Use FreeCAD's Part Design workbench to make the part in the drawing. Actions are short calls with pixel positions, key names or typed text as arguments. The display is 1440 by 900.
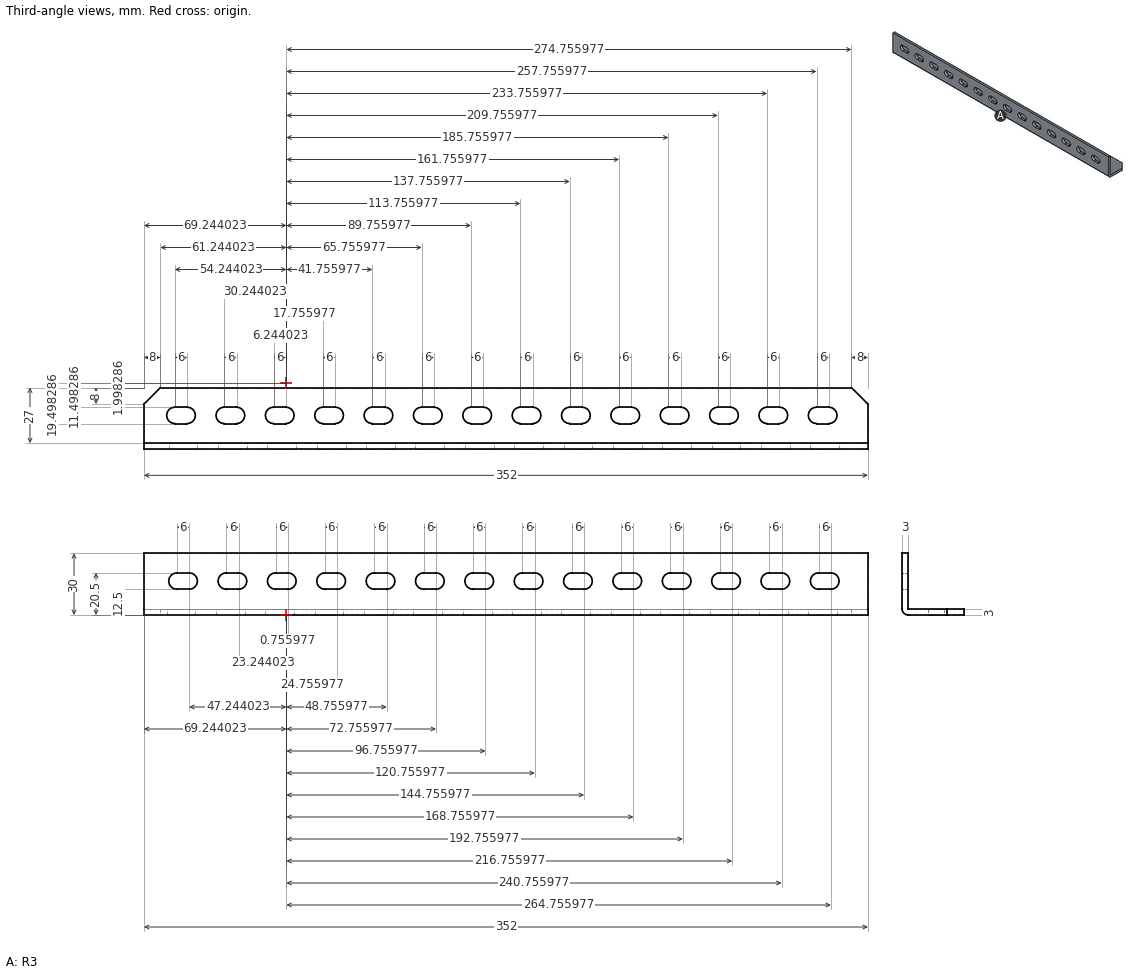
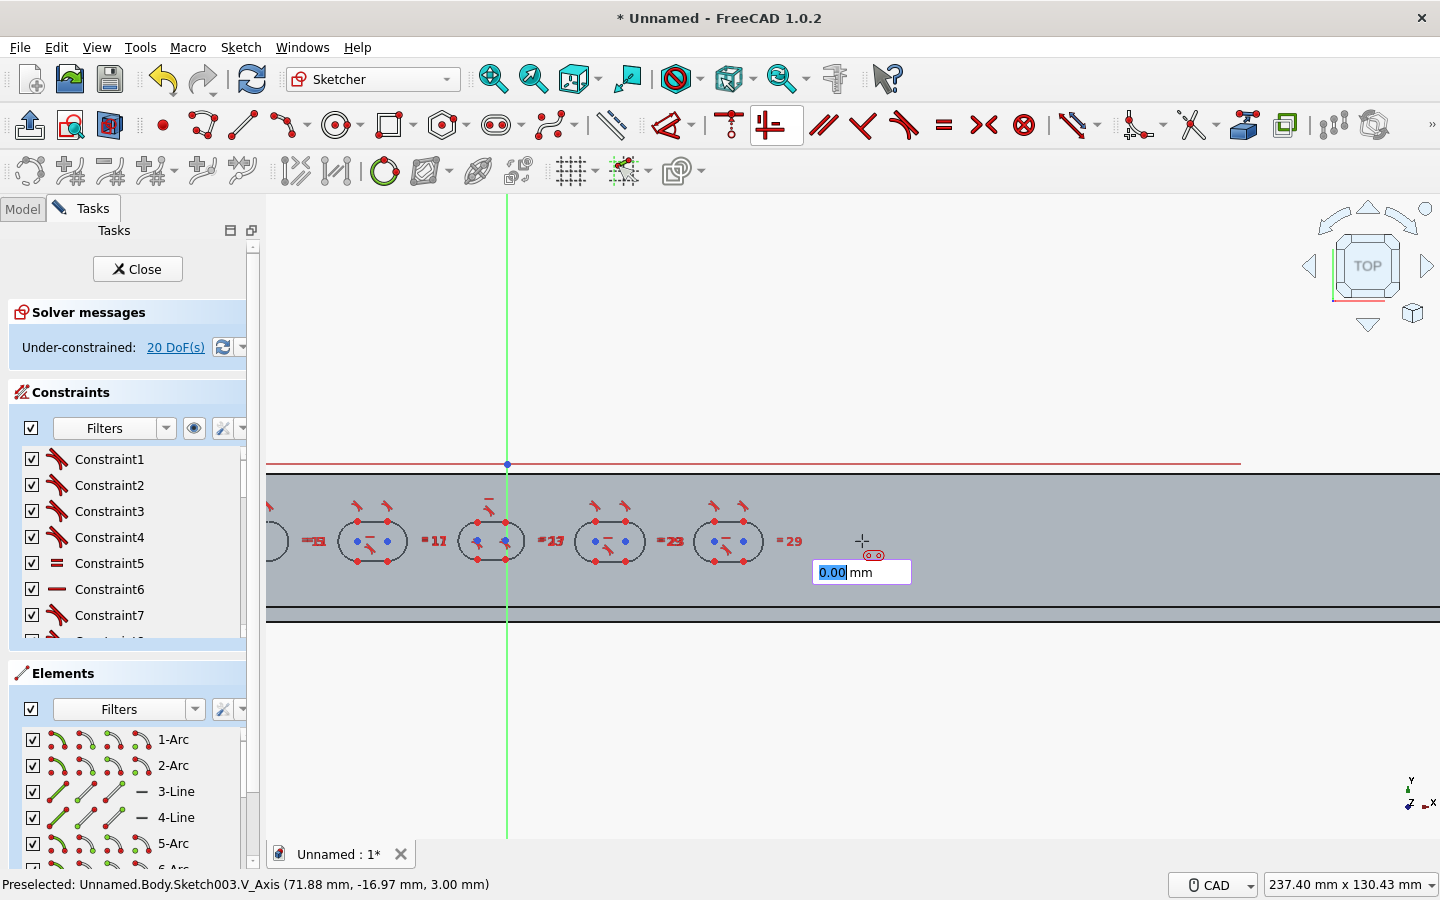
click(847, 521)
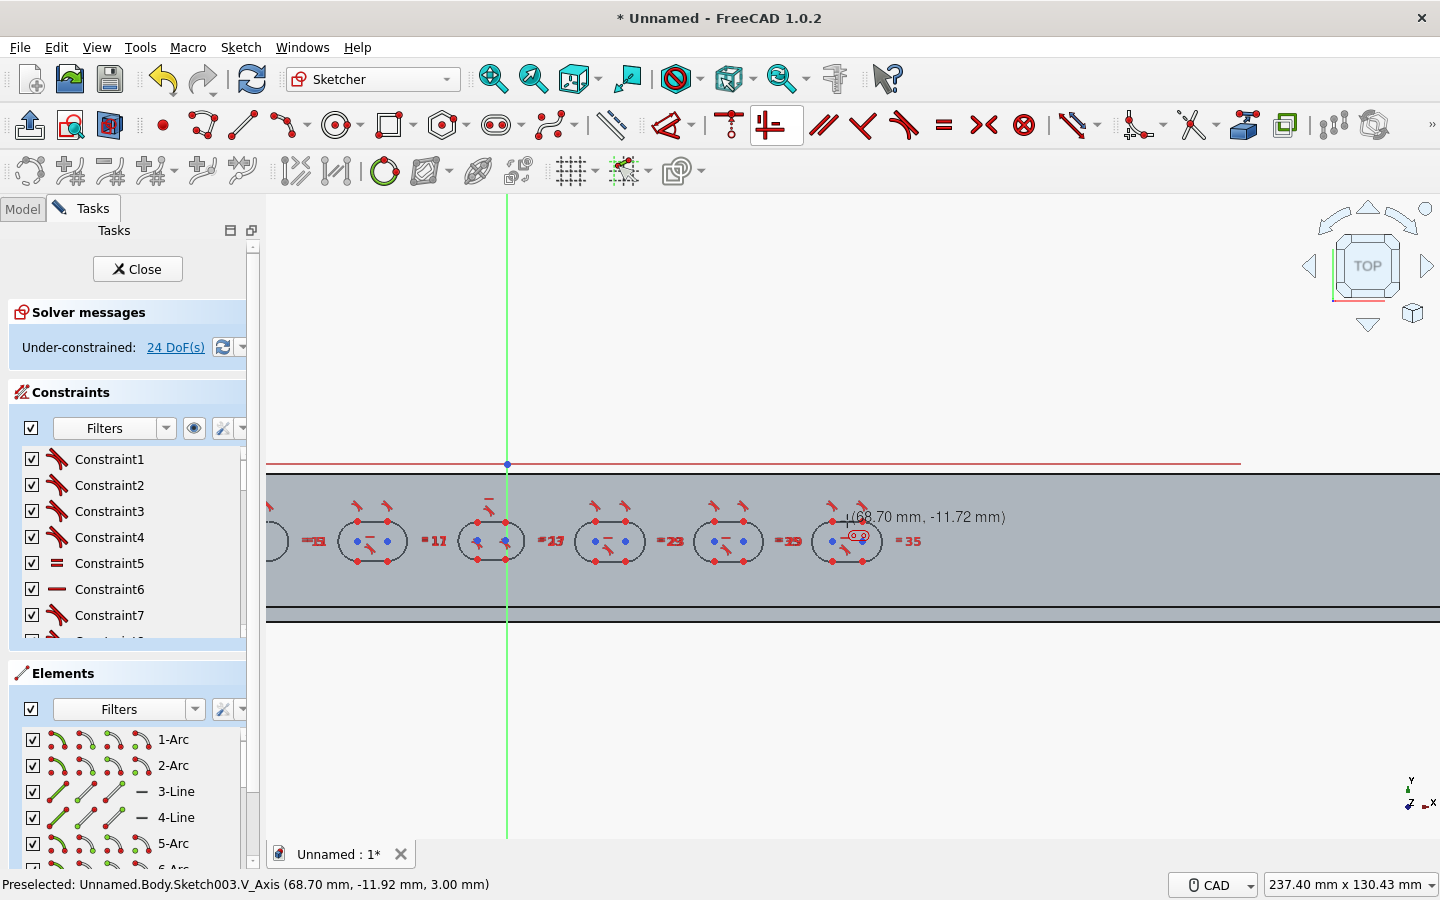
click(951, 541)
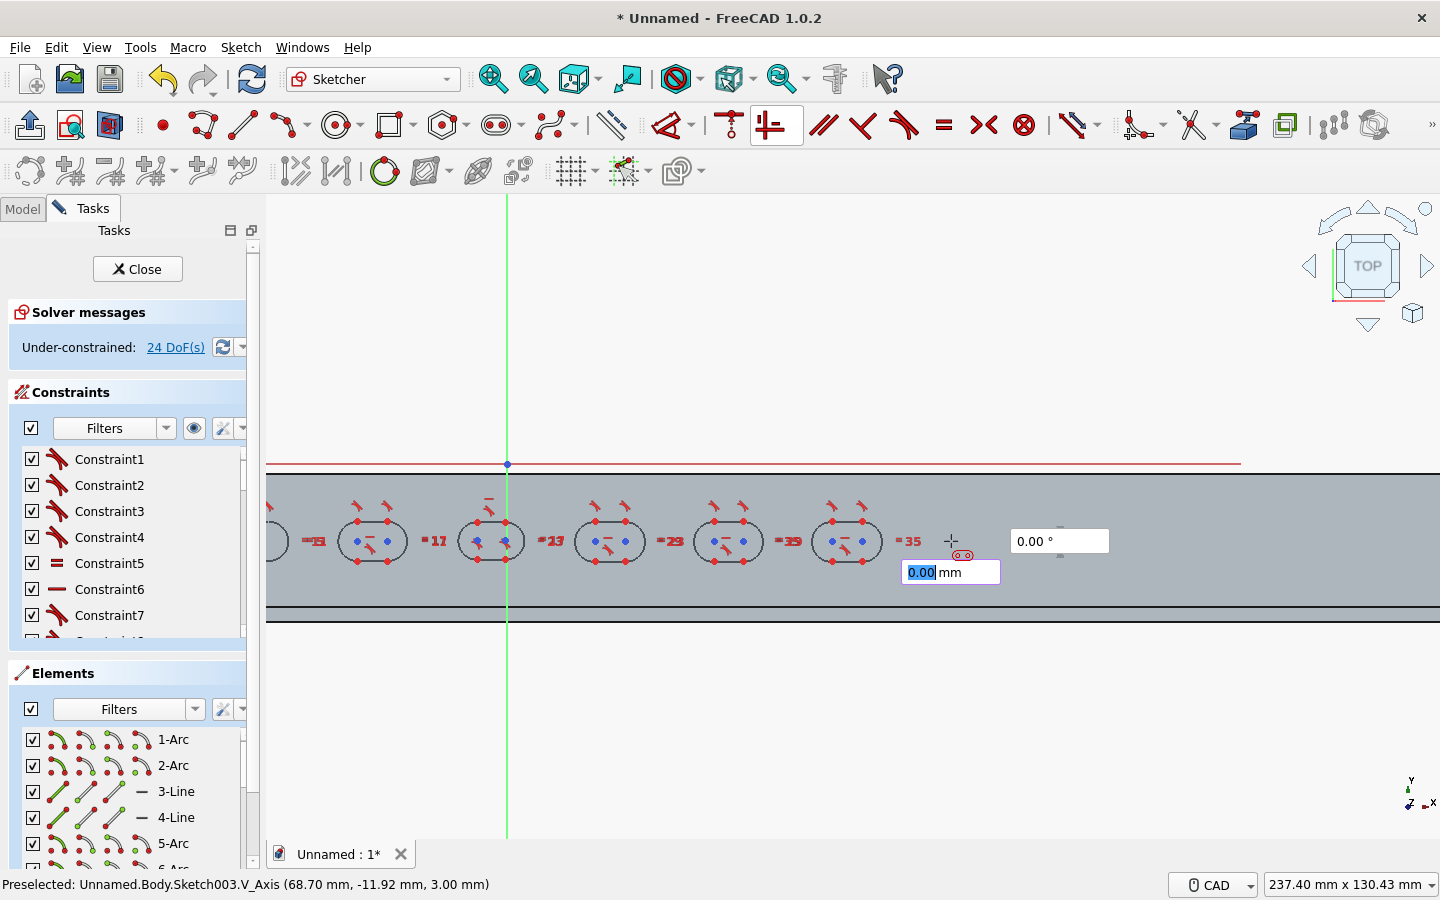
click(981, 541)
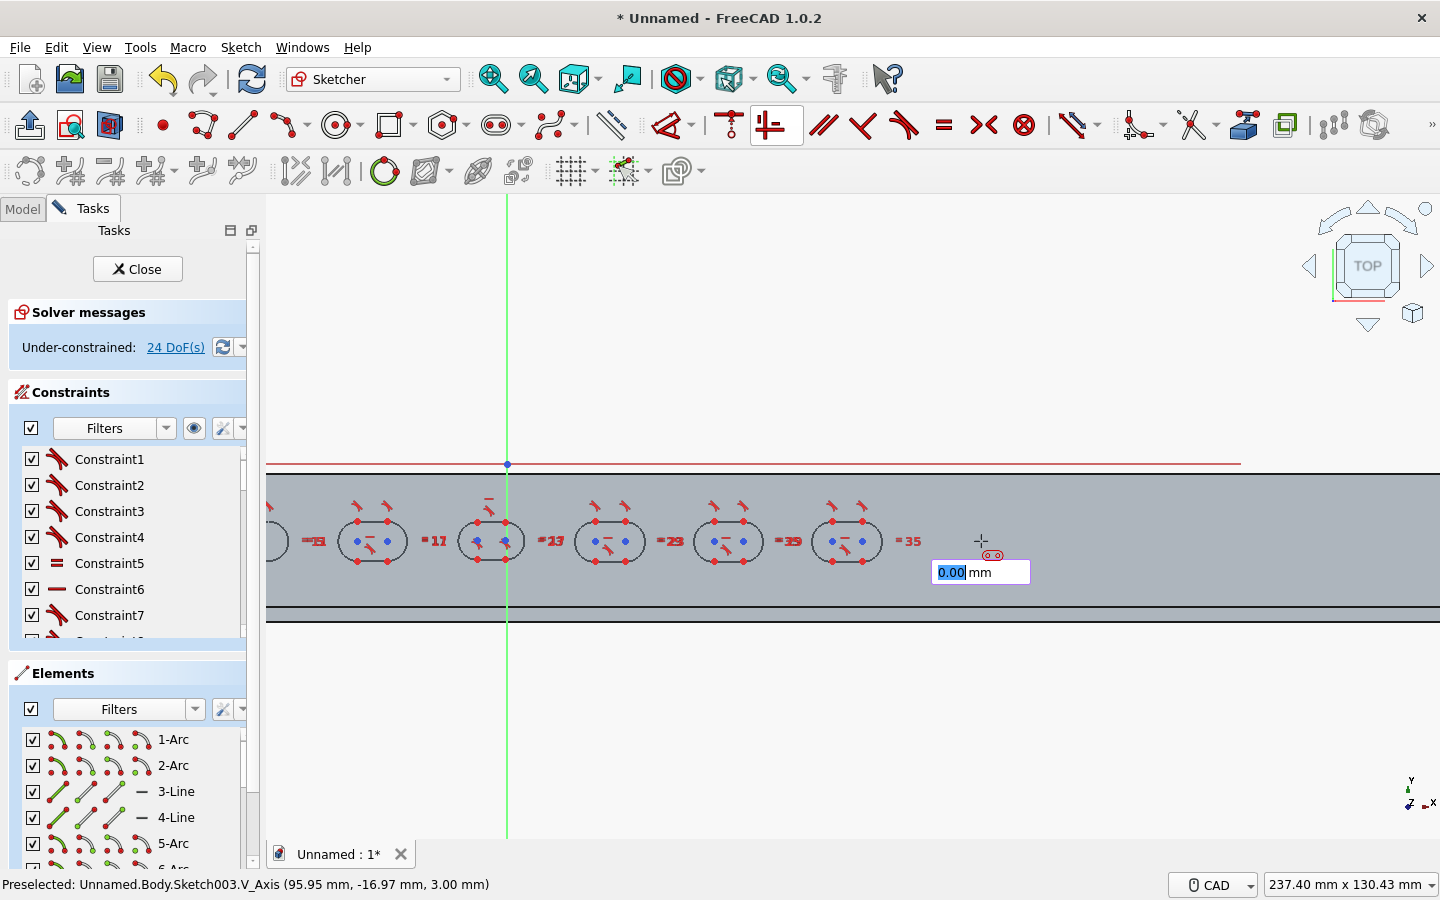
click(966, 521)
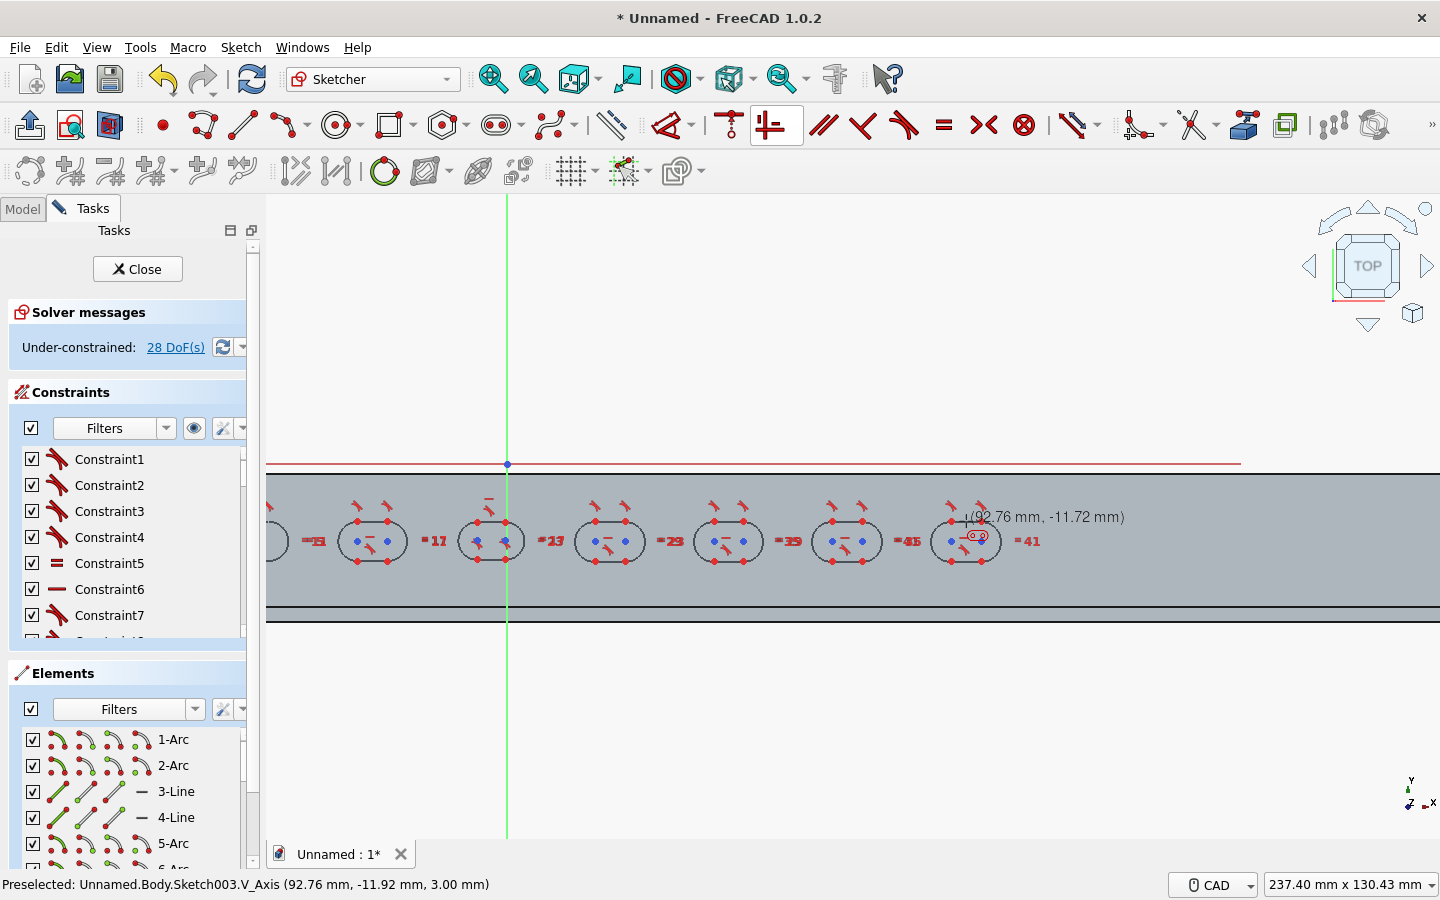
click(1070, 541)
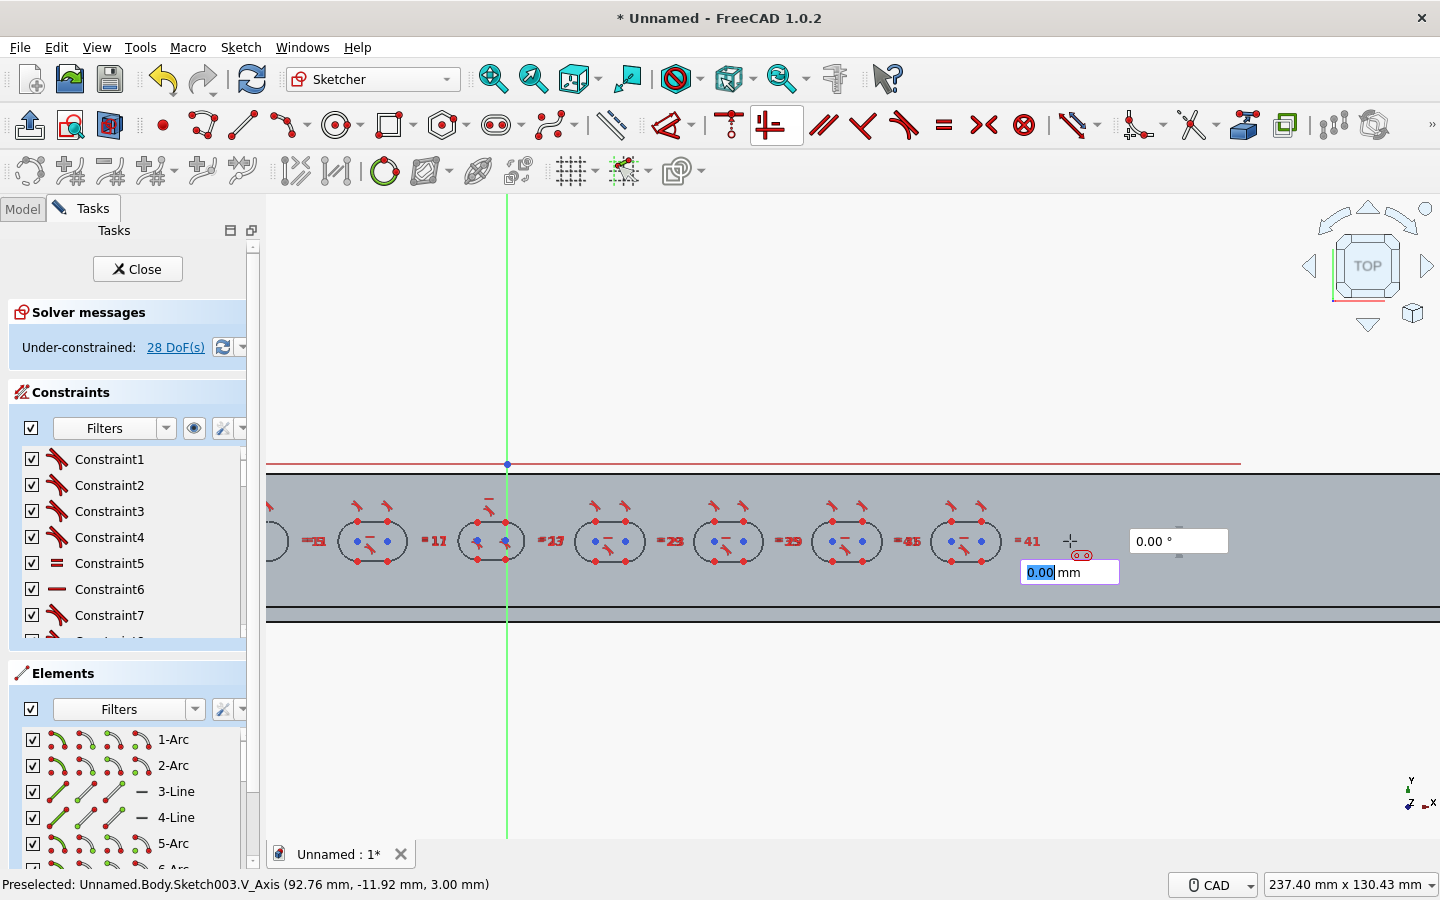
click(1099, 541)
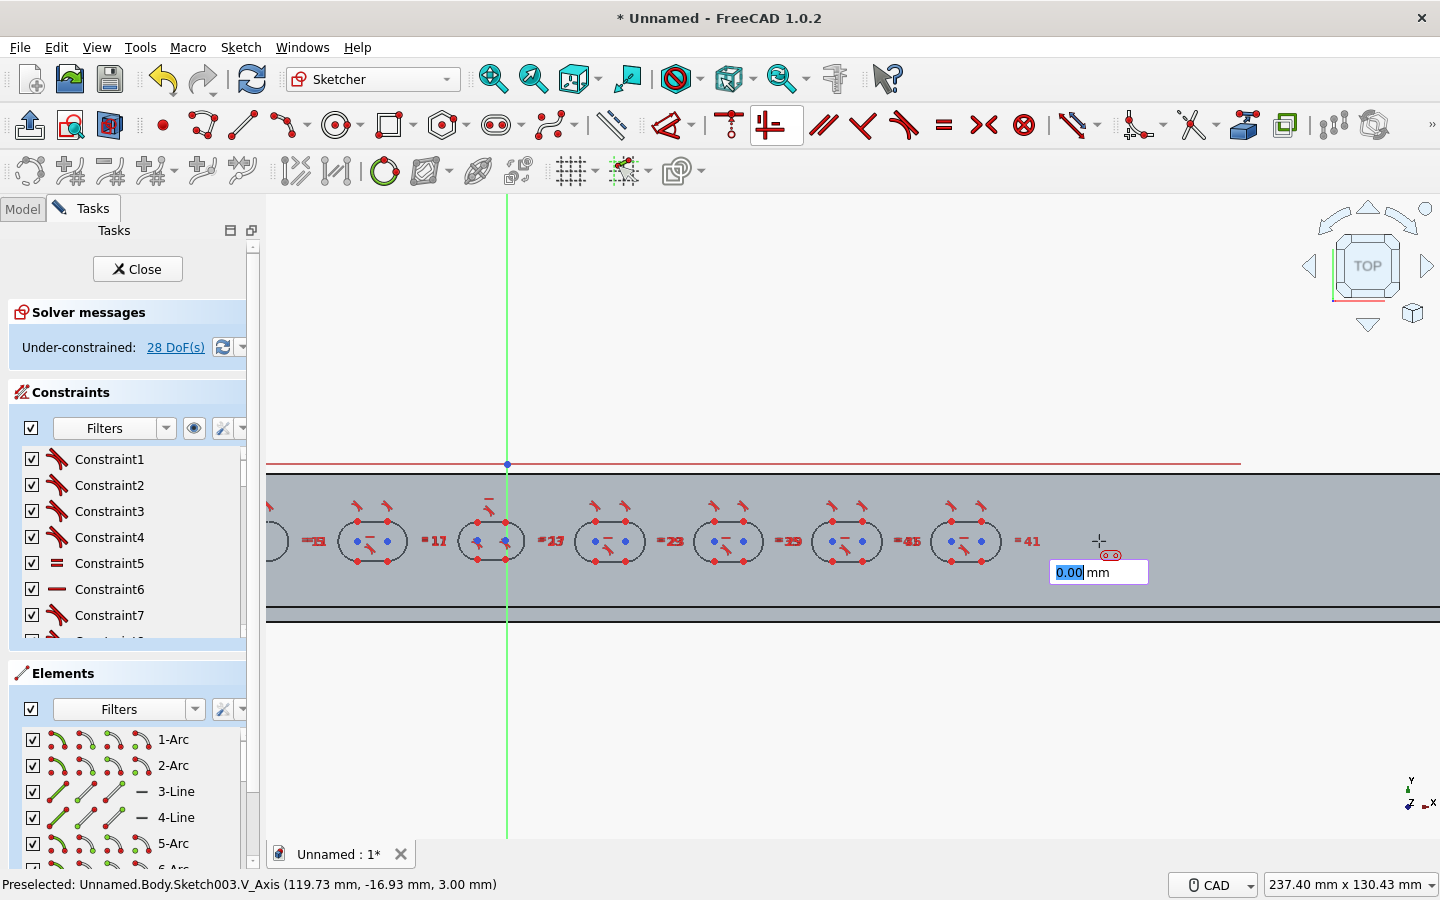
click(1085, 521)